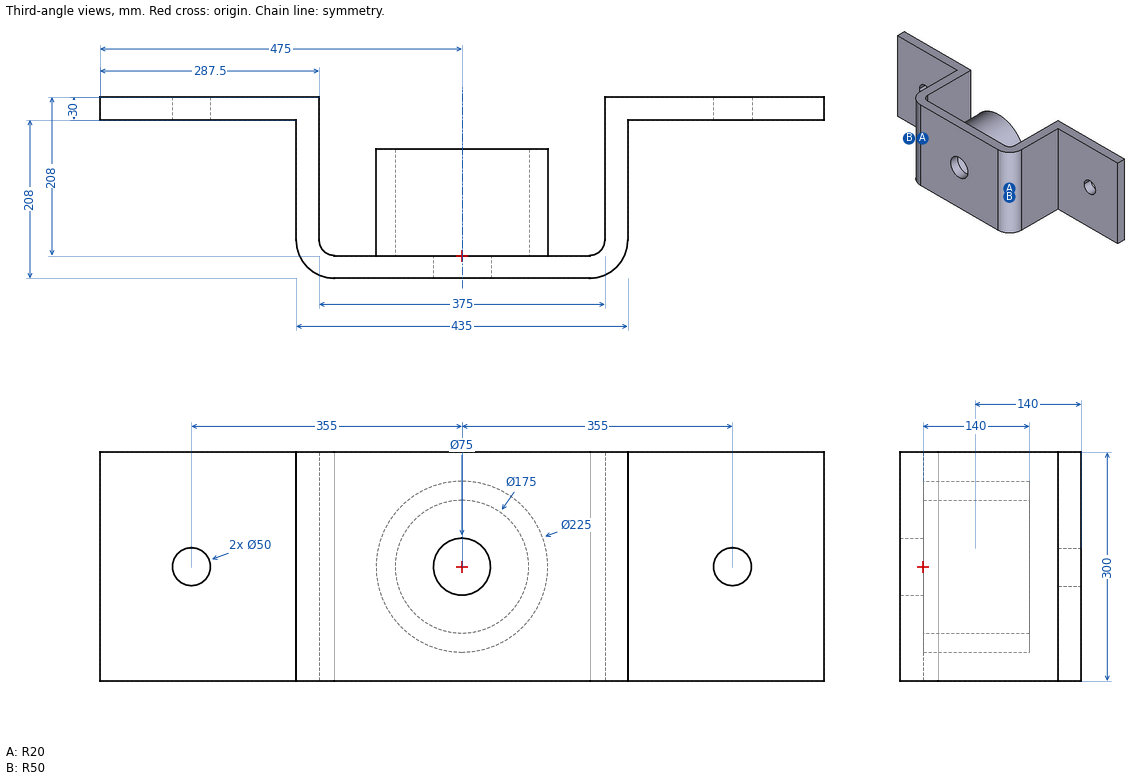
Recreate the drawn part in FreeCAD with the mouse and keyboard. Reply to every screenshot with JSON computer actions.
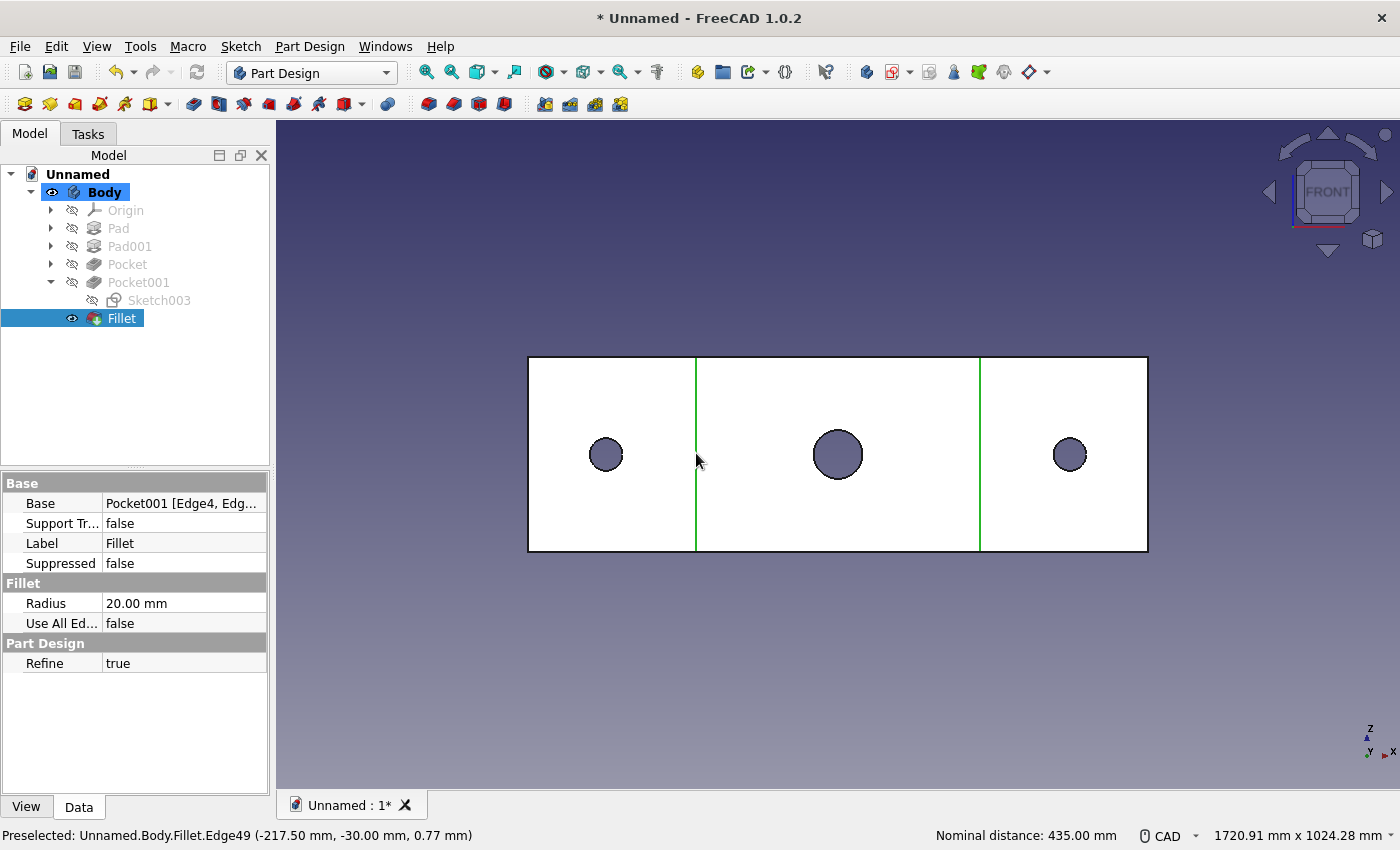
{"action": "left_click", "coordinate": [429, 104]}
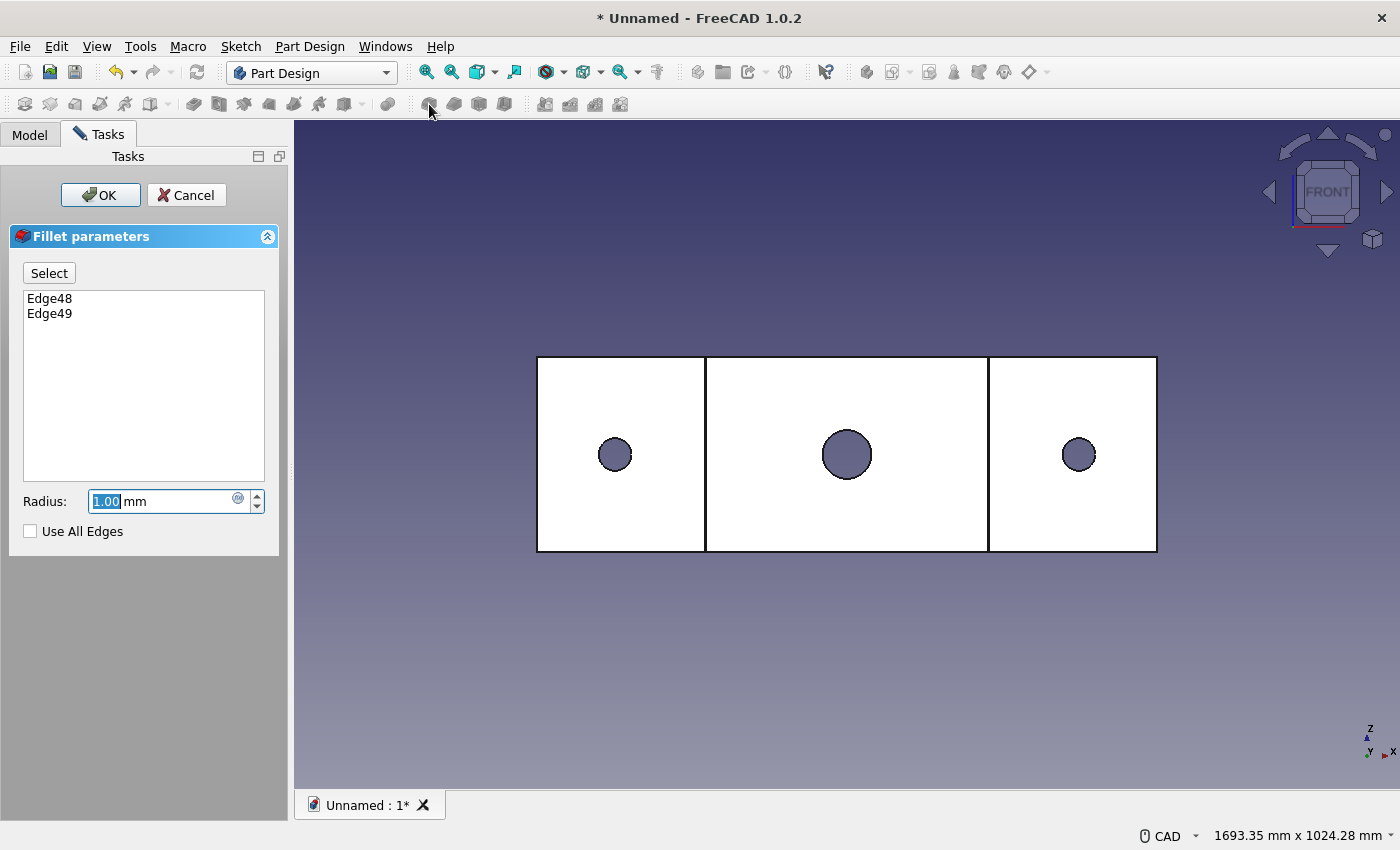
{"action": "type", "text": "50"}
{"action": "key", "text": "Tab"}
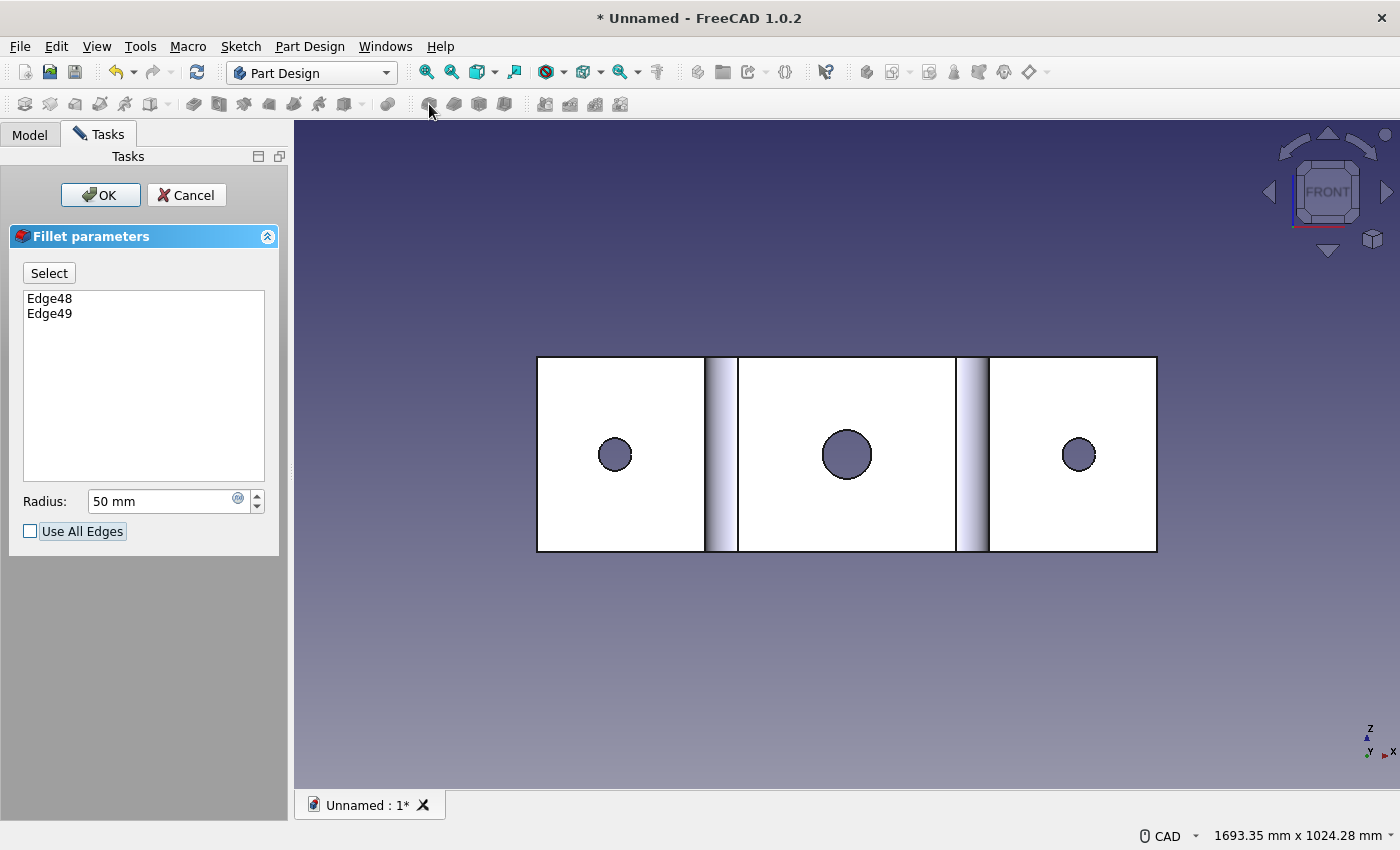
{"action": "left_click", "coordinate": [101, 195]}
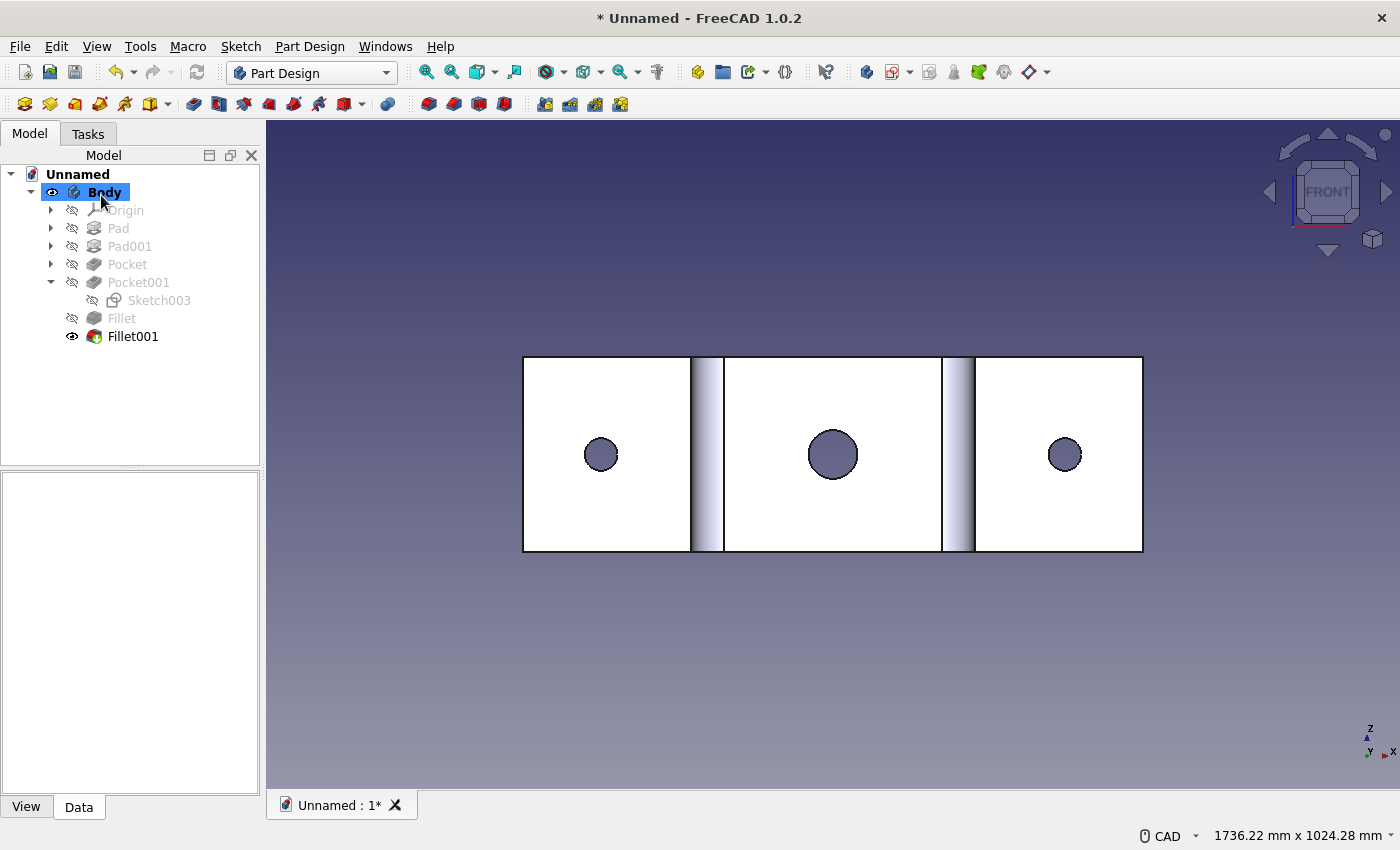
{"action": "key", "text": "0"}